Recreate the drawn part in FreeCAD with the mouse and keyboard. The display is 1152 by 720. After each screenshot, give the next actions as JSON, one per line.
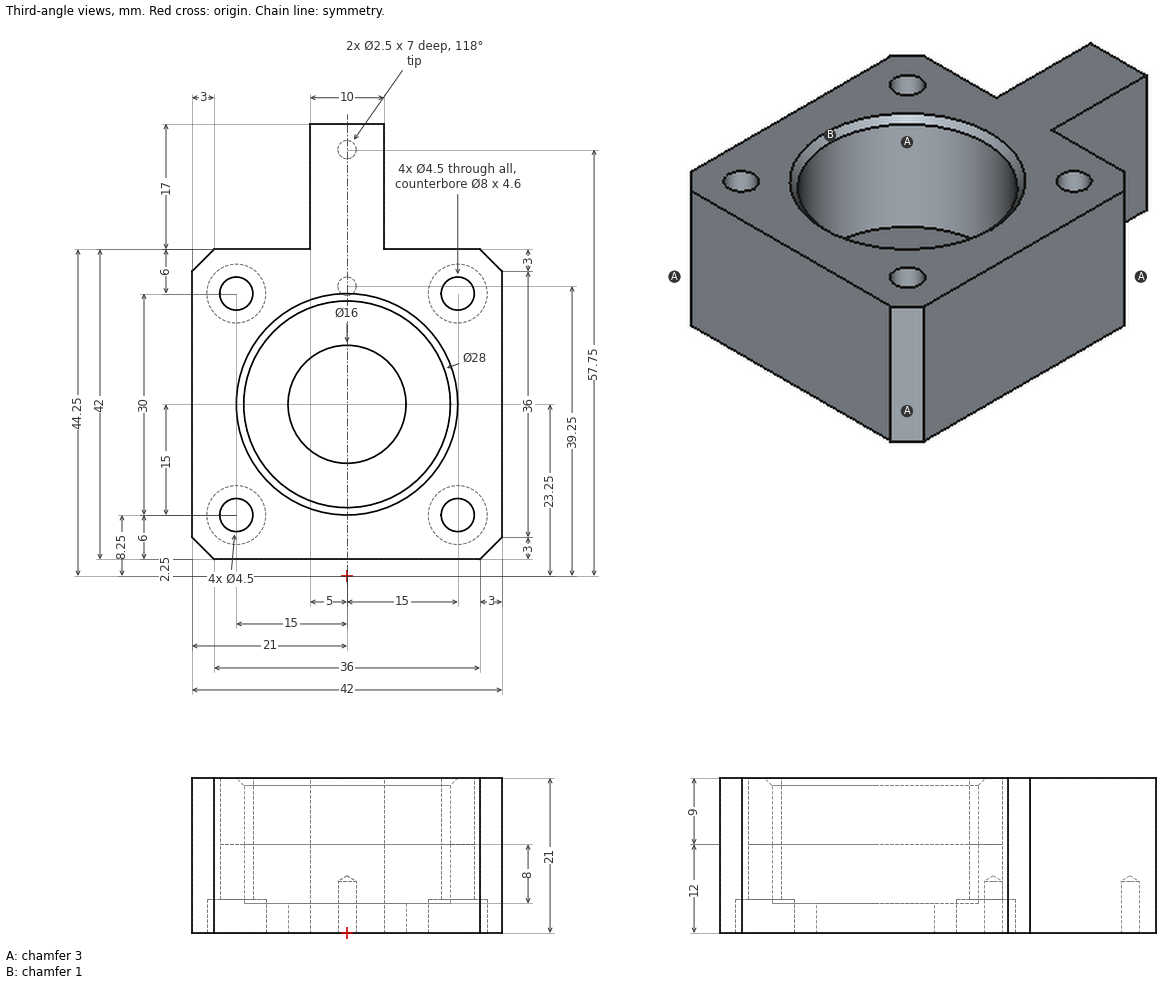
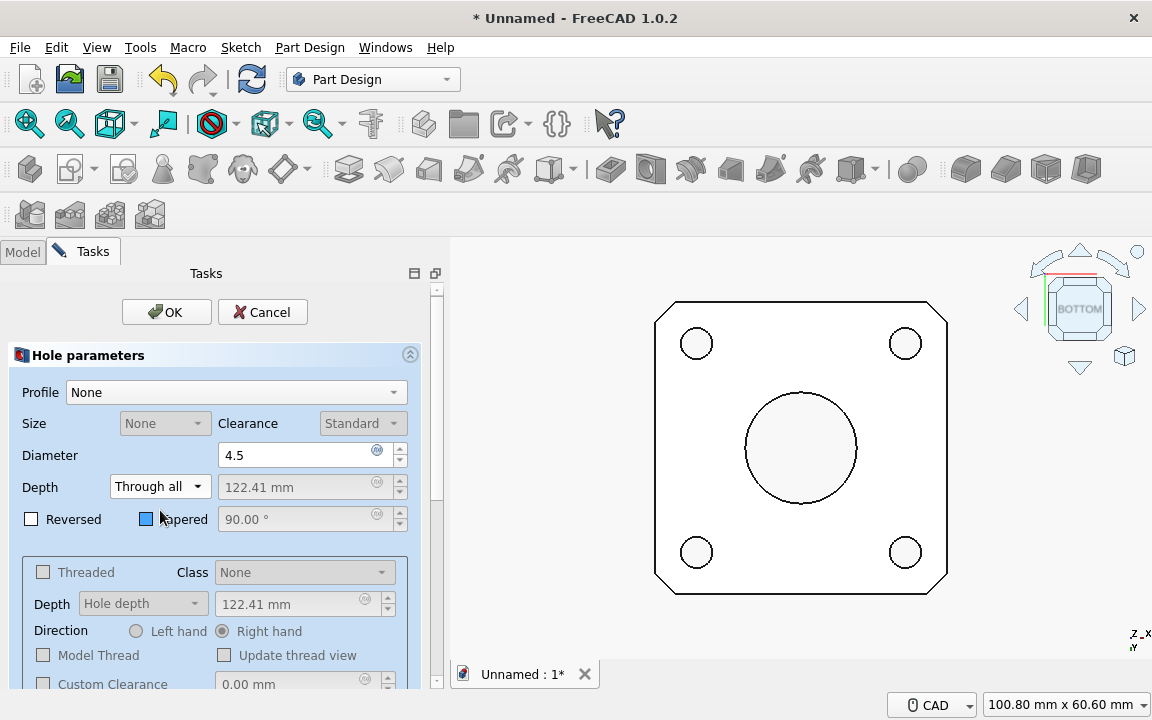
{"action": "scroll", "coordinate": [437, 486], "scroll_direction": "down", "scroll_amount": 3}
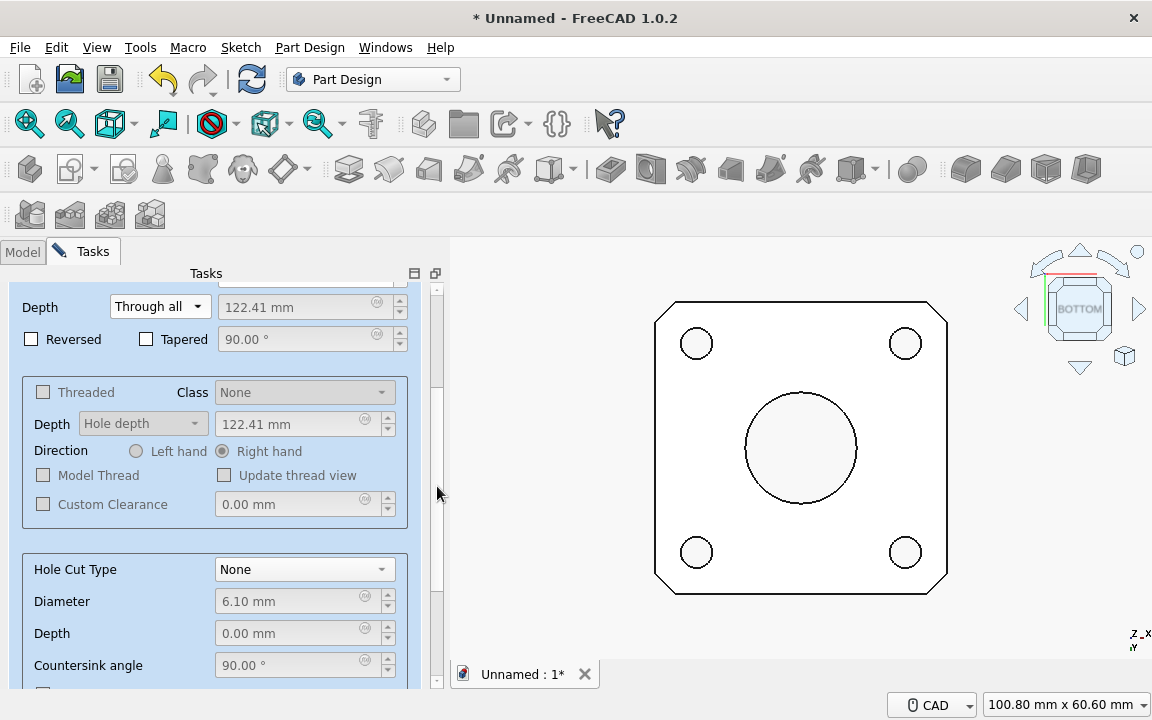
{"action": "left_click", "coordinate": [306, 570]}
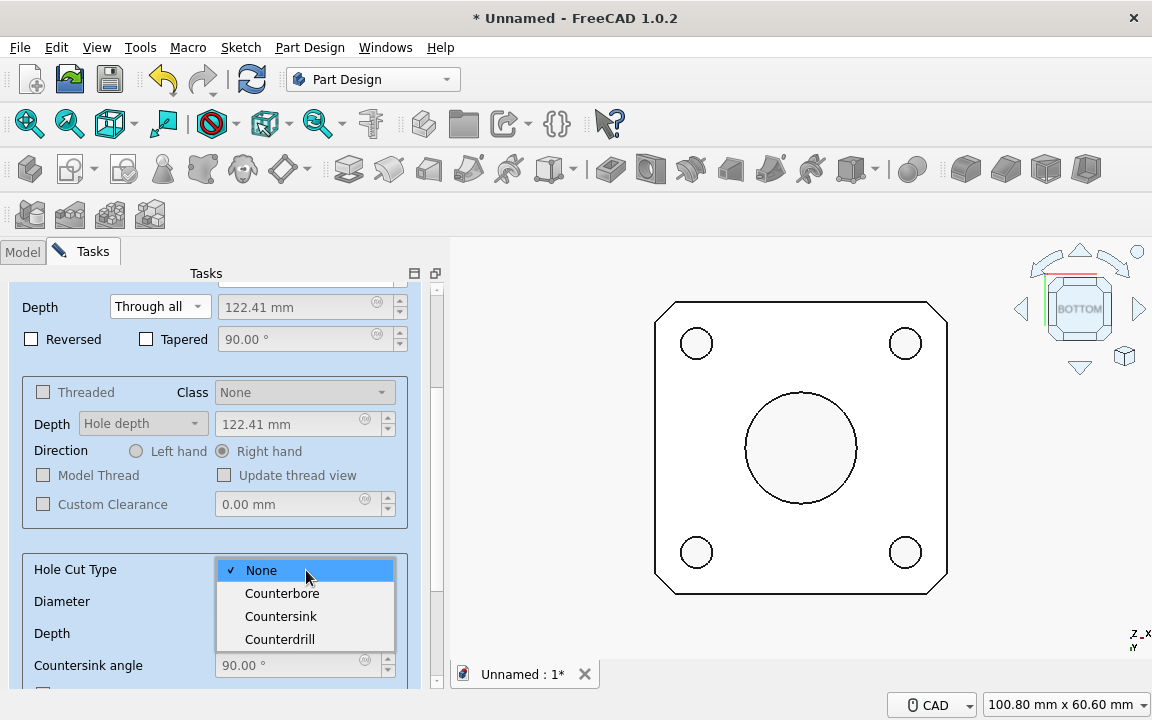
{"action": "left_click", "coordinate": [304, 594]}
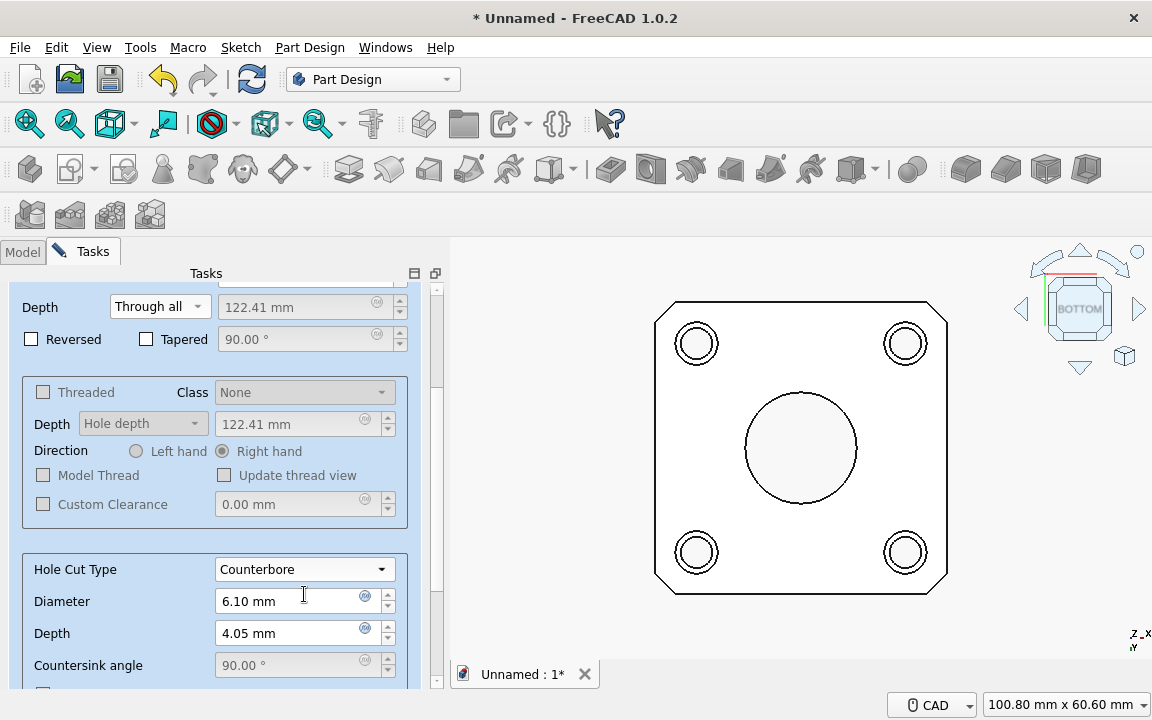
{"action": "triple_click", "coordinate": [298, 601]}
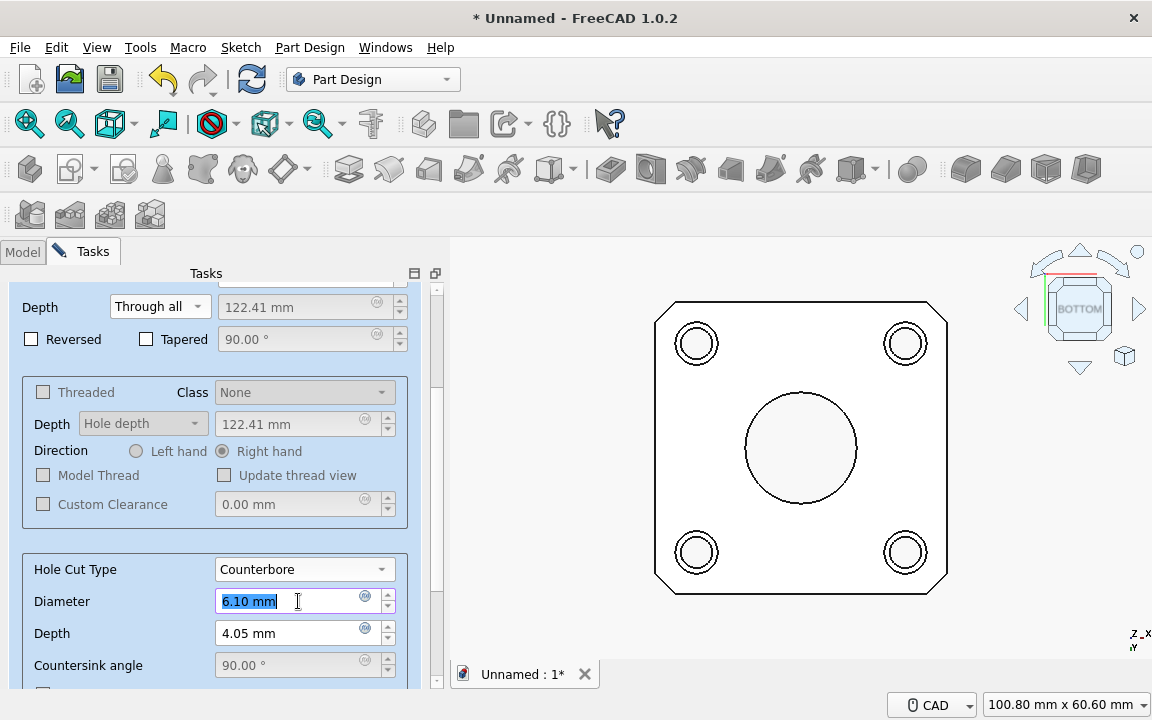
{"action": "type", "text": "8"}
{"action": "key", "text": "Tab"}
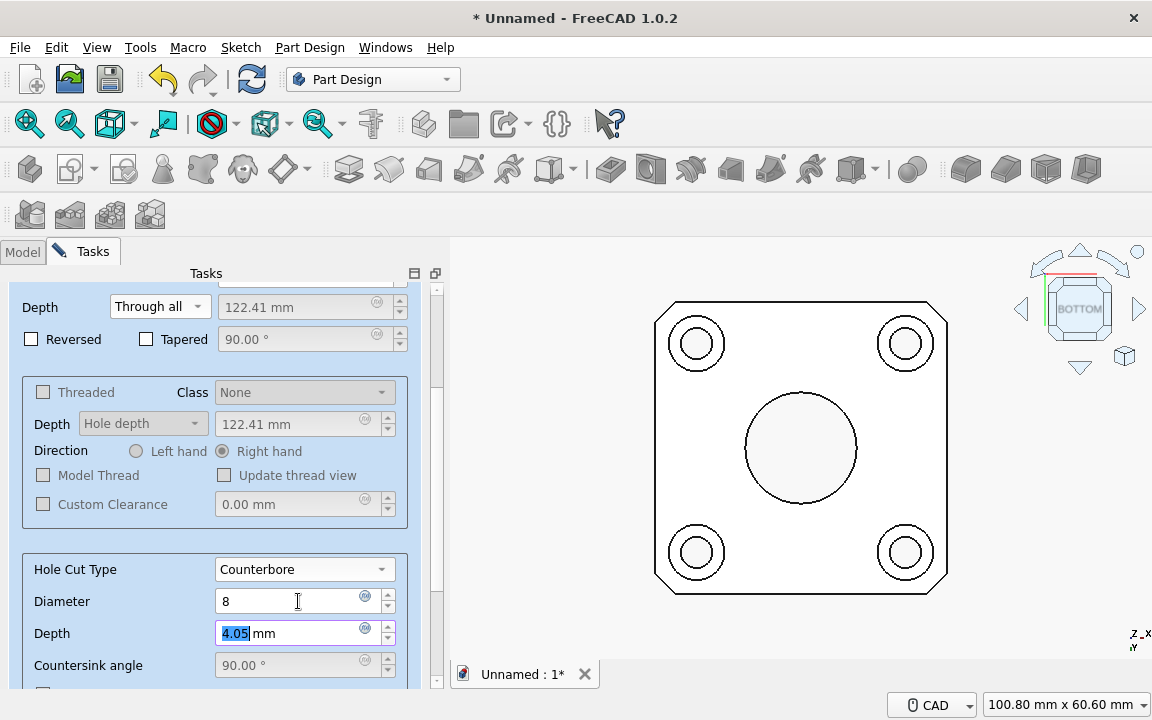
{"action": "type", "text": "4.6"}
{"action": "key", "text": "Tab"}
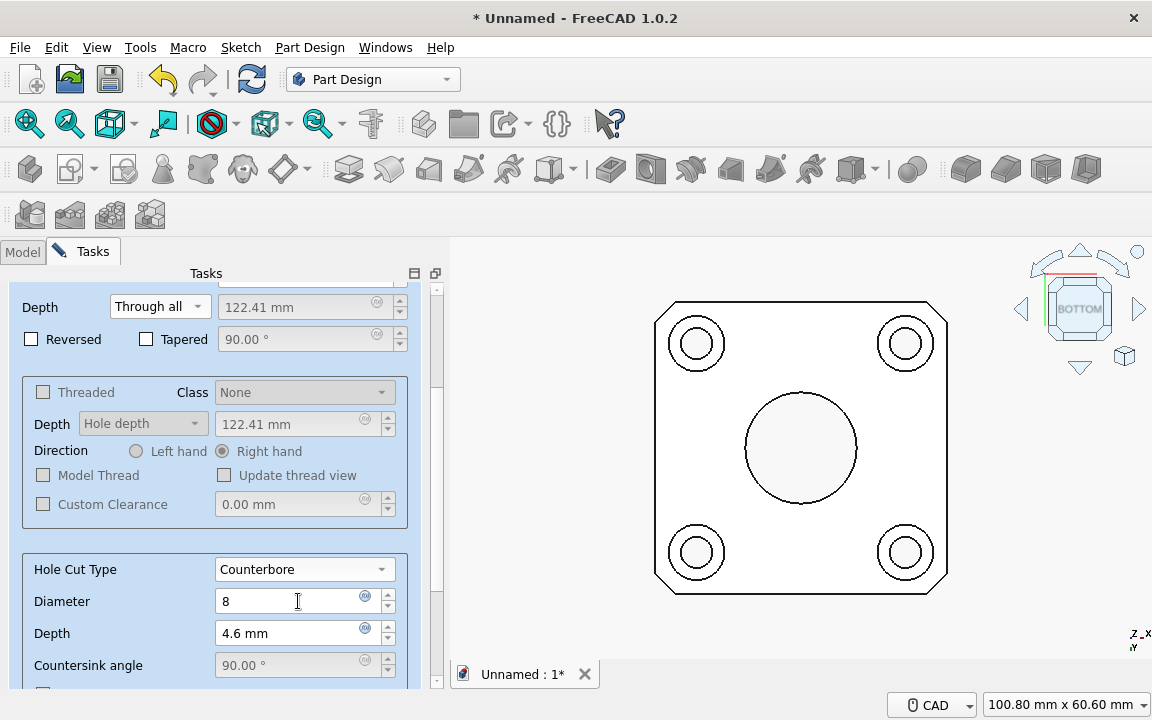
{"action": "scroll", "coordinate": [437, 486], "scroll_direction": "up", "scroll_amount": 4}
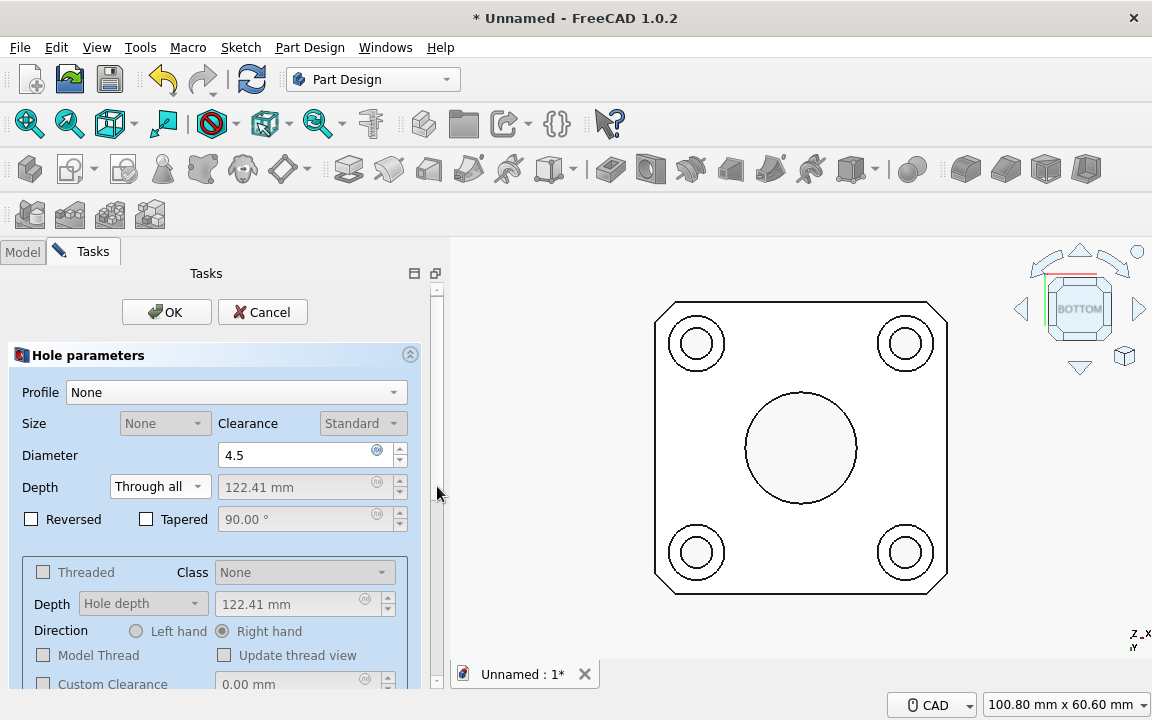
{"action": "left_click", "coordinate": [167, 312]}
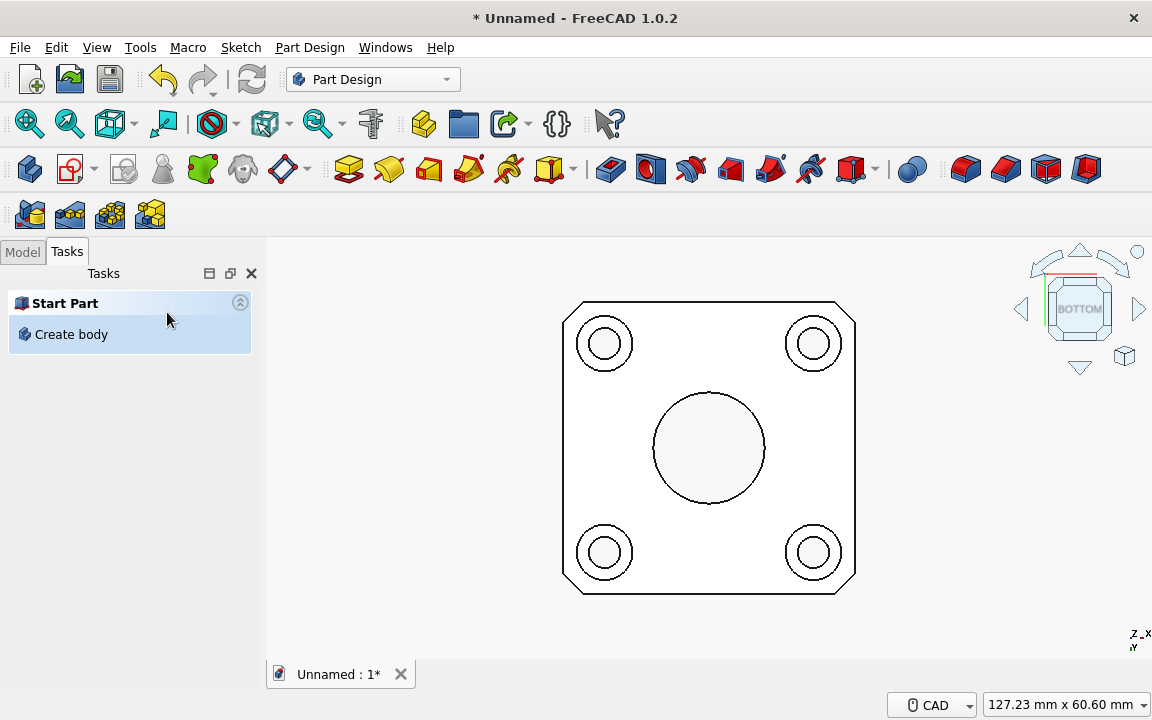
{"action": "left_click", "coordinate": [23, 251]}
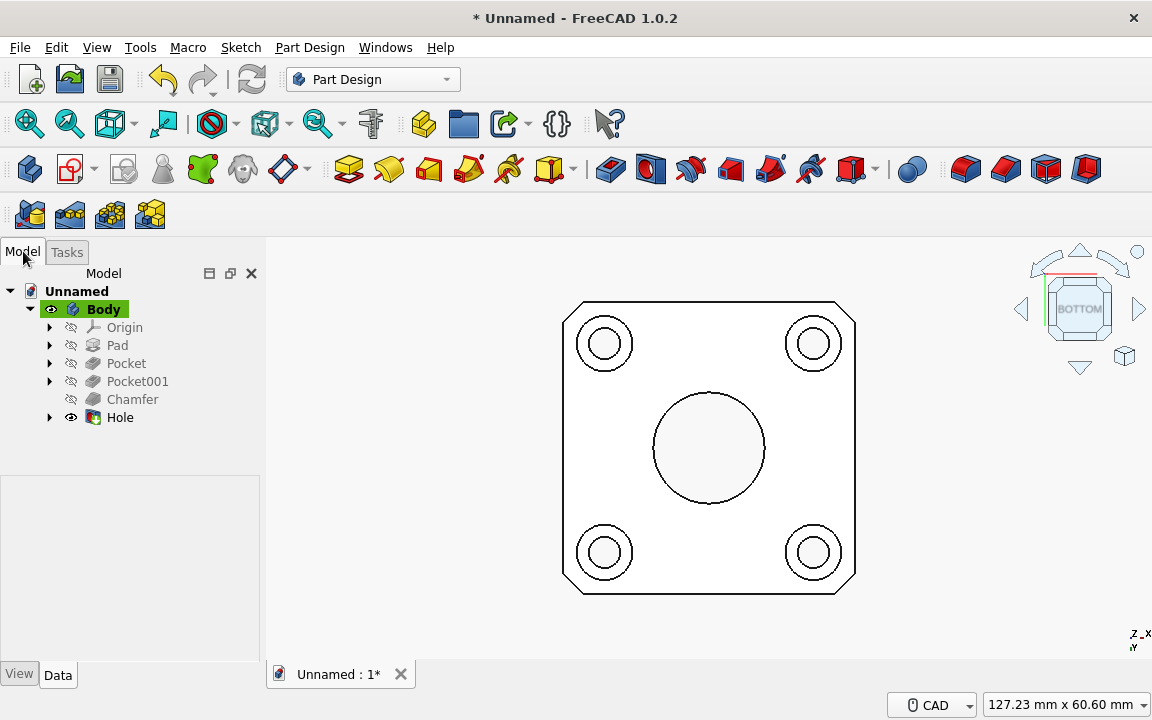
{"action": "left_click", "coordinate": [50, 327]}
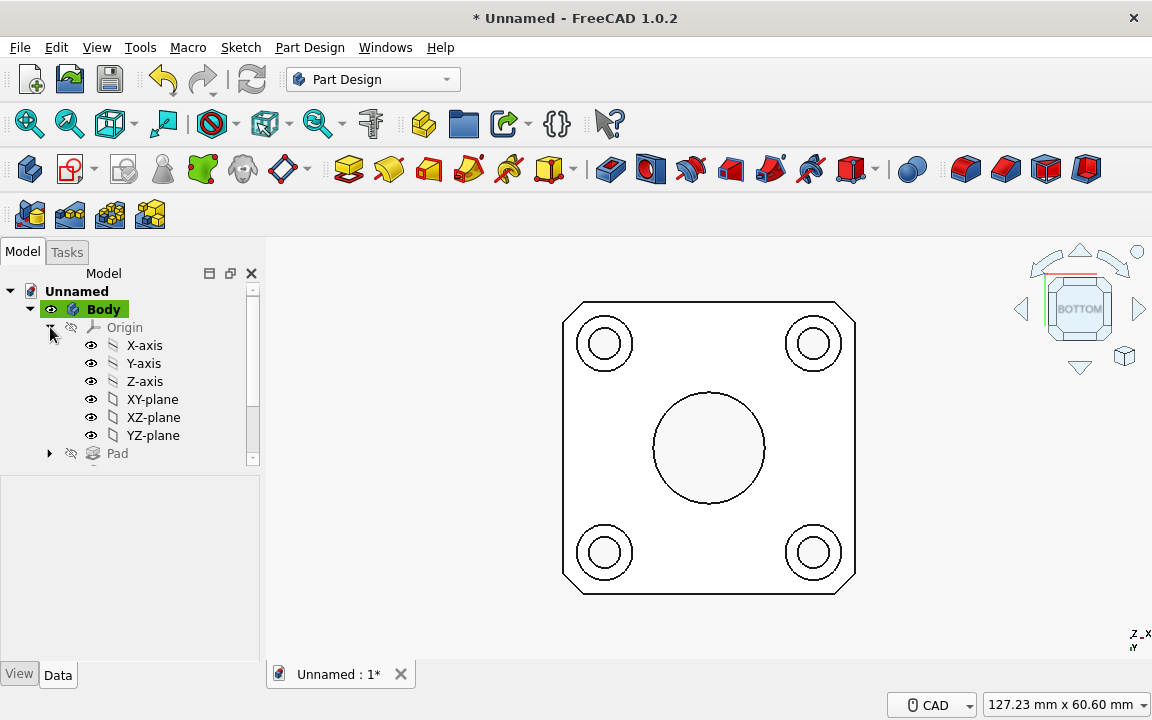
{"action": "left_click", "coordinate": [136, 399]}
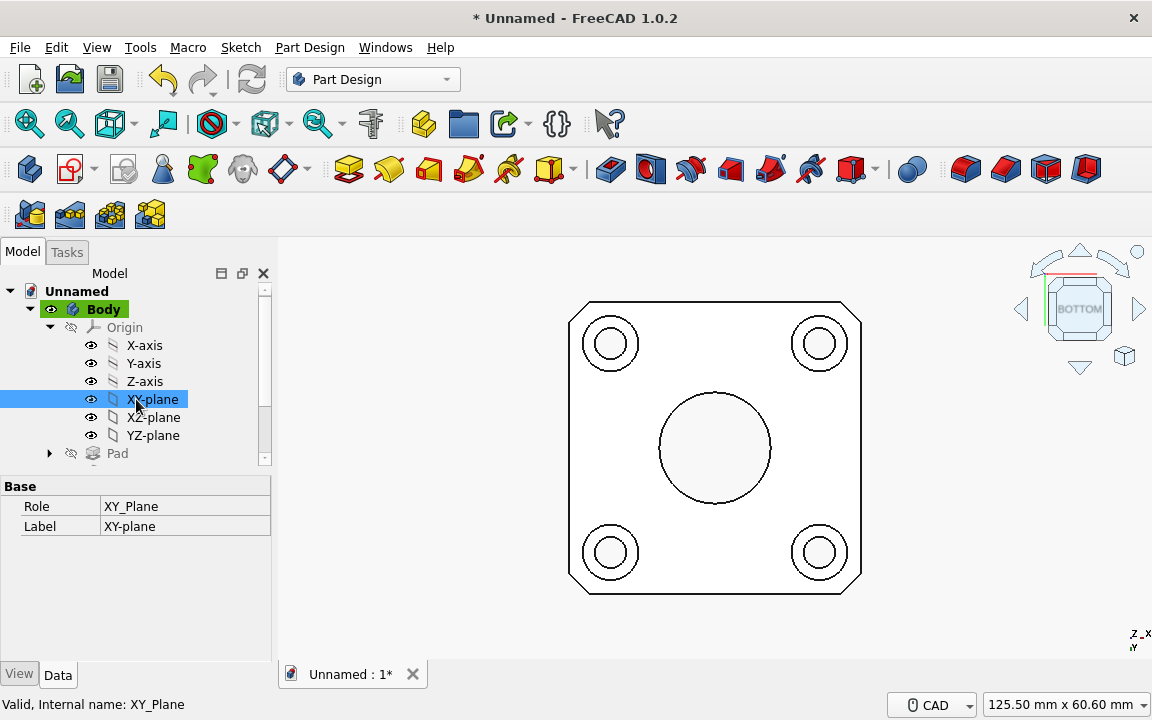
{"action": "left_click", "coordinate": [284, 170]}